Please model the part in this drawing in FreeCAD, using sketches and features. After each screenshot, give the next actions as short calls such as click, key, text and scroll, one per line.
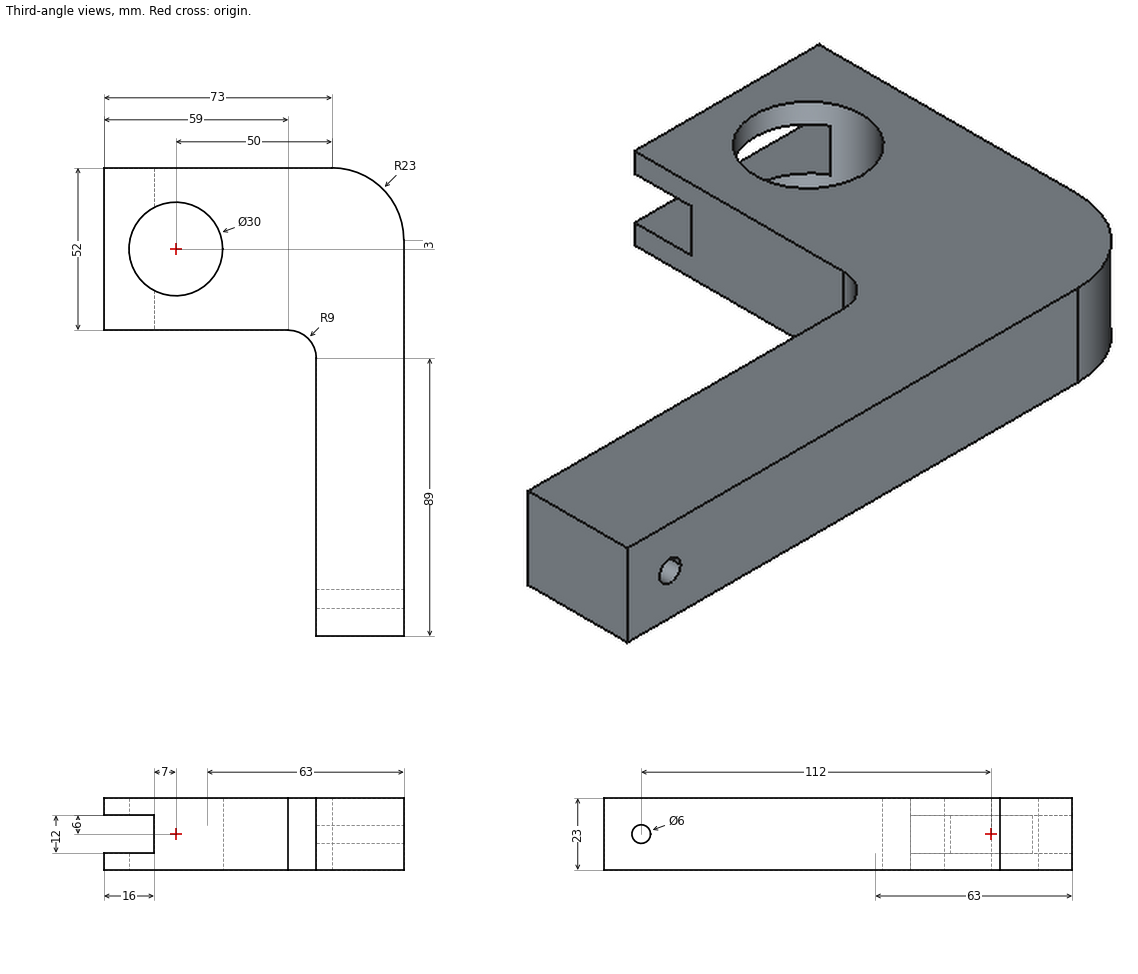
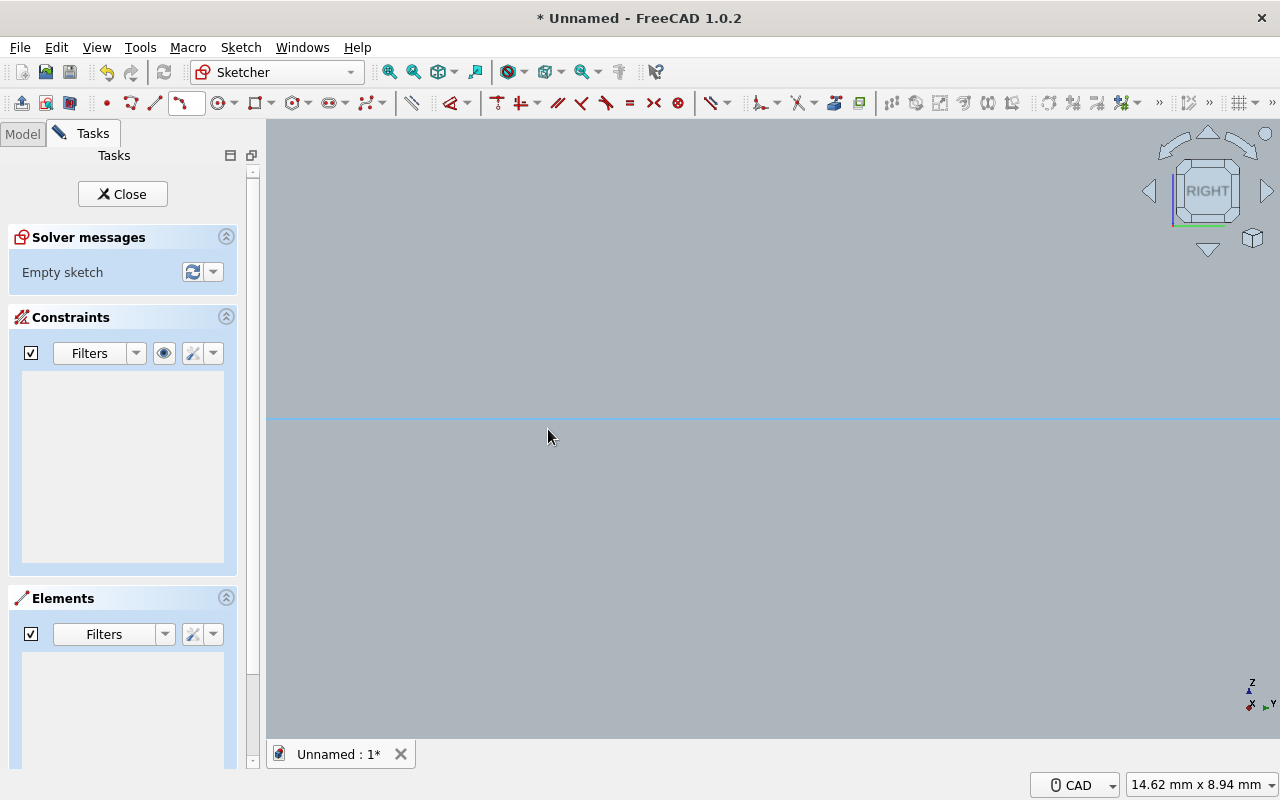
click(218, 104)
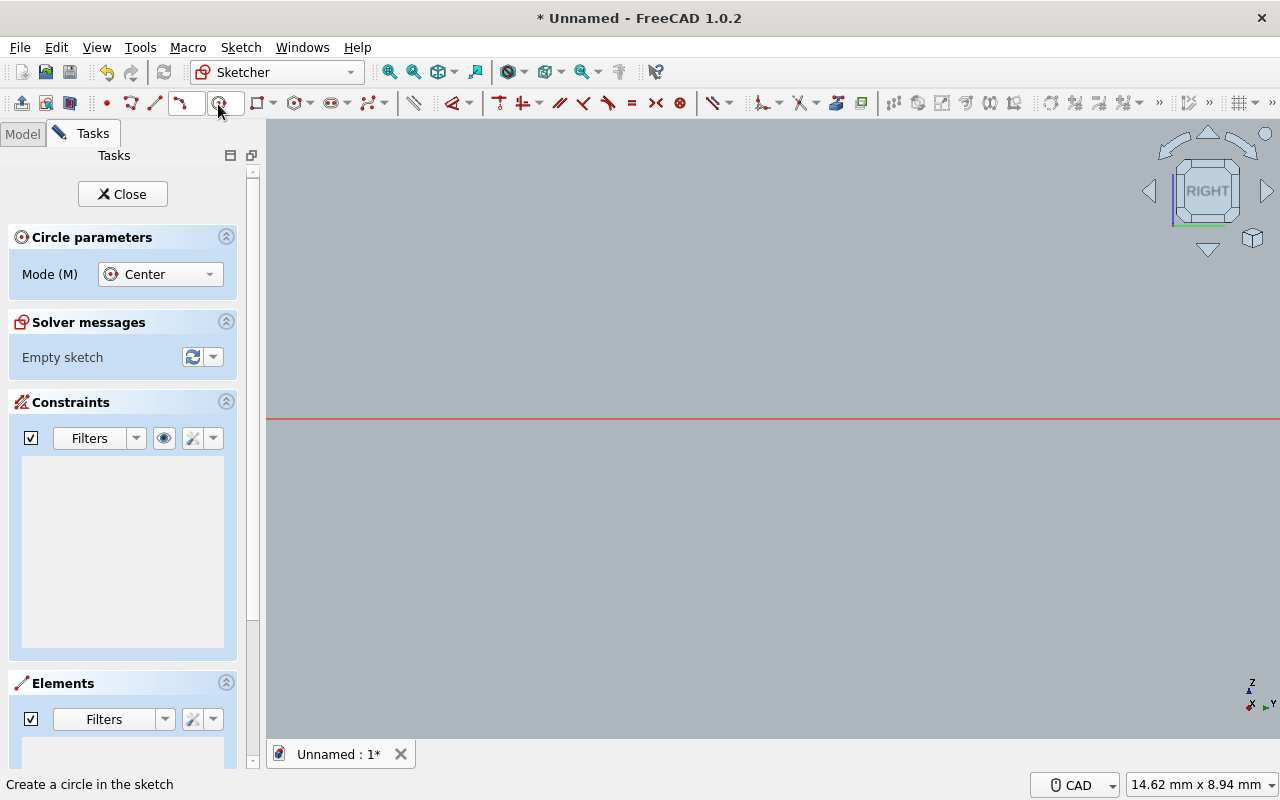
click(693, 419)
move(840, 272)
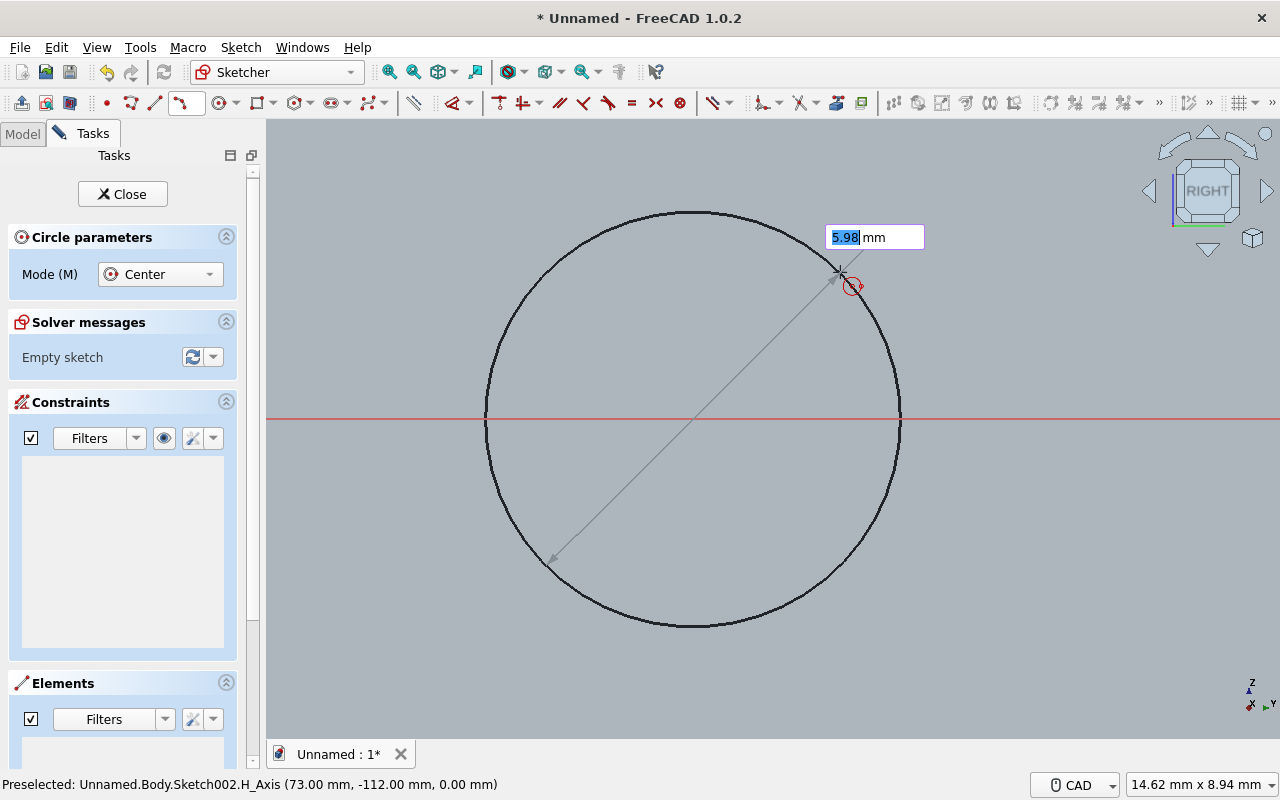
text(6)
key(Return)
key(Escape)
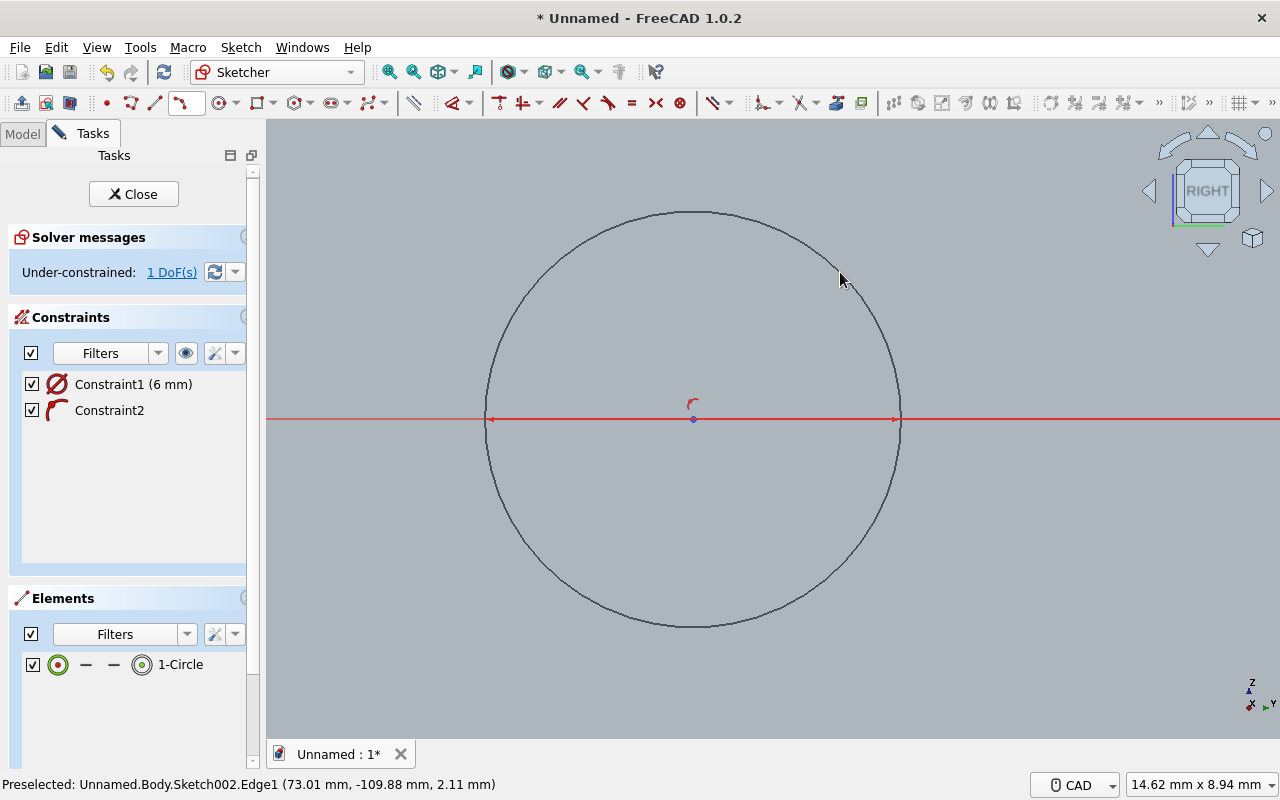
click(452, 104)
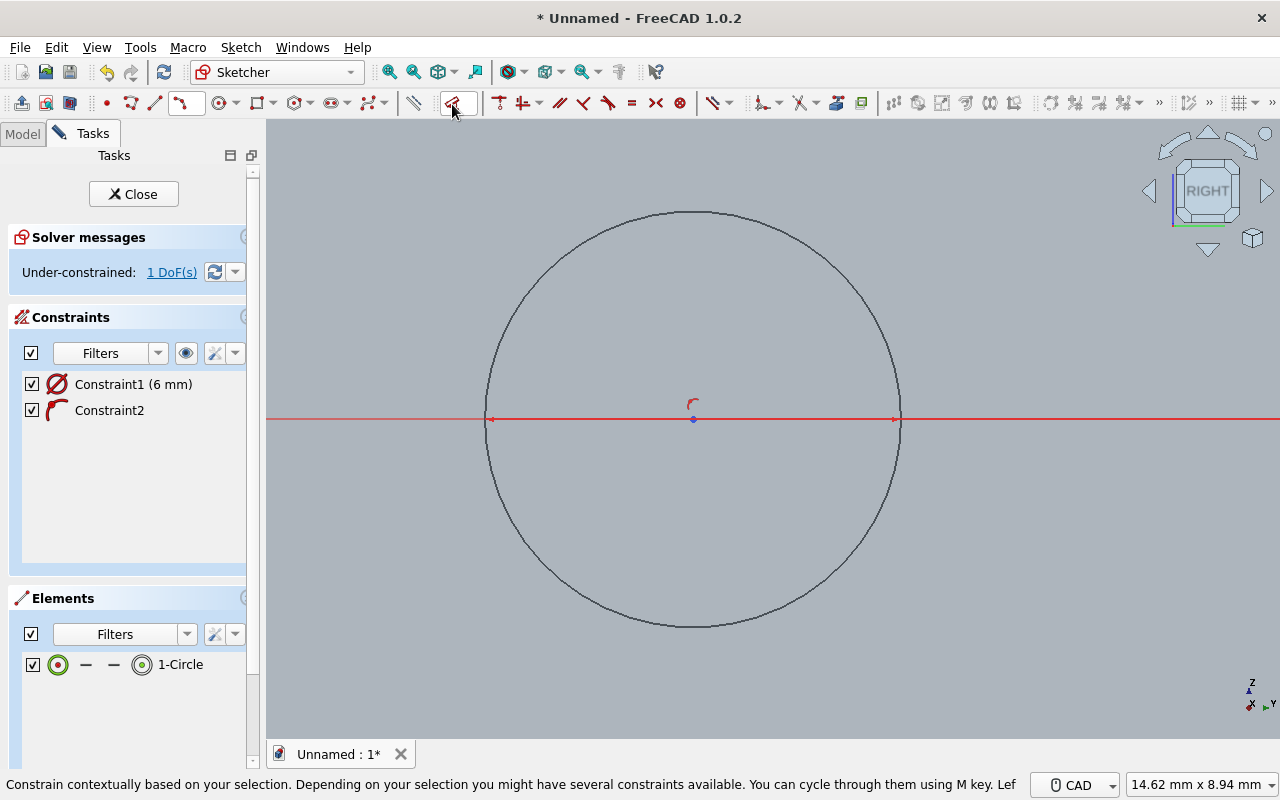
click(693, 419)
click(807, 453)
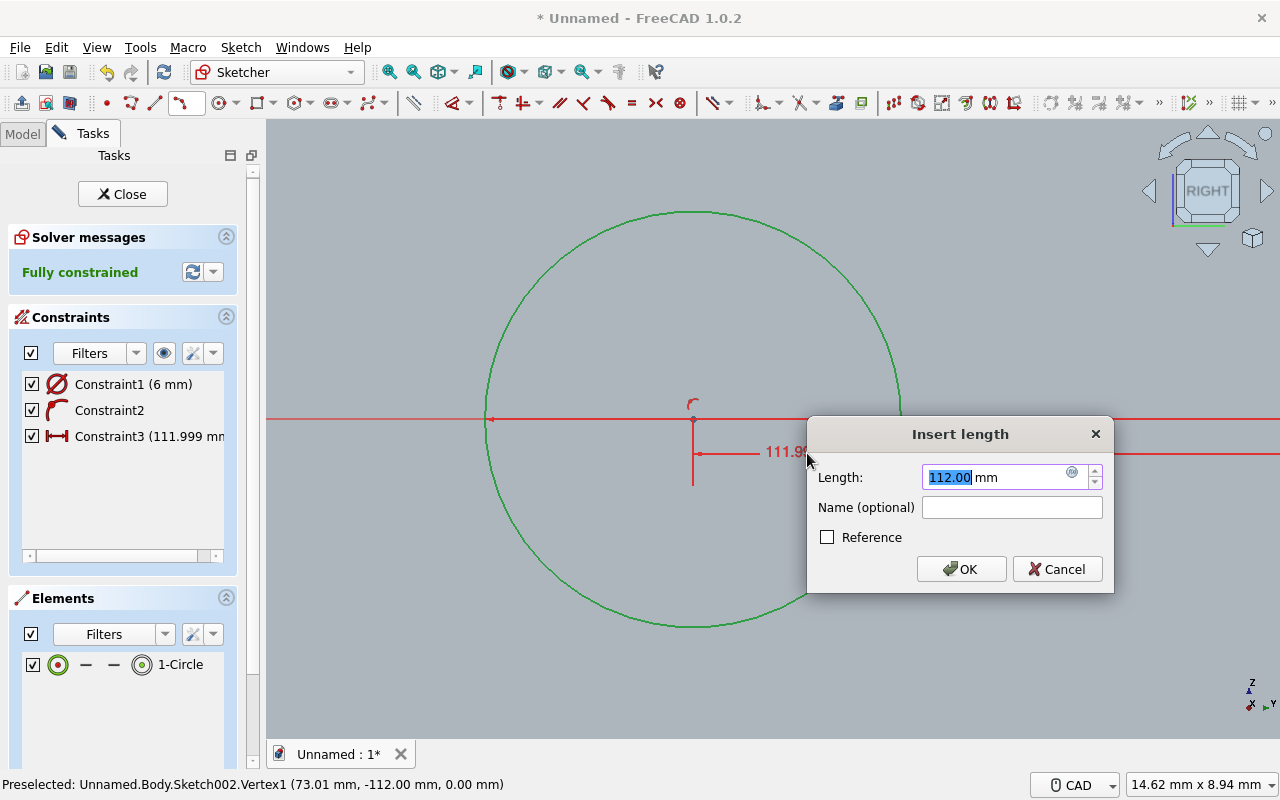
text(112)
key(Return)
key(Escape)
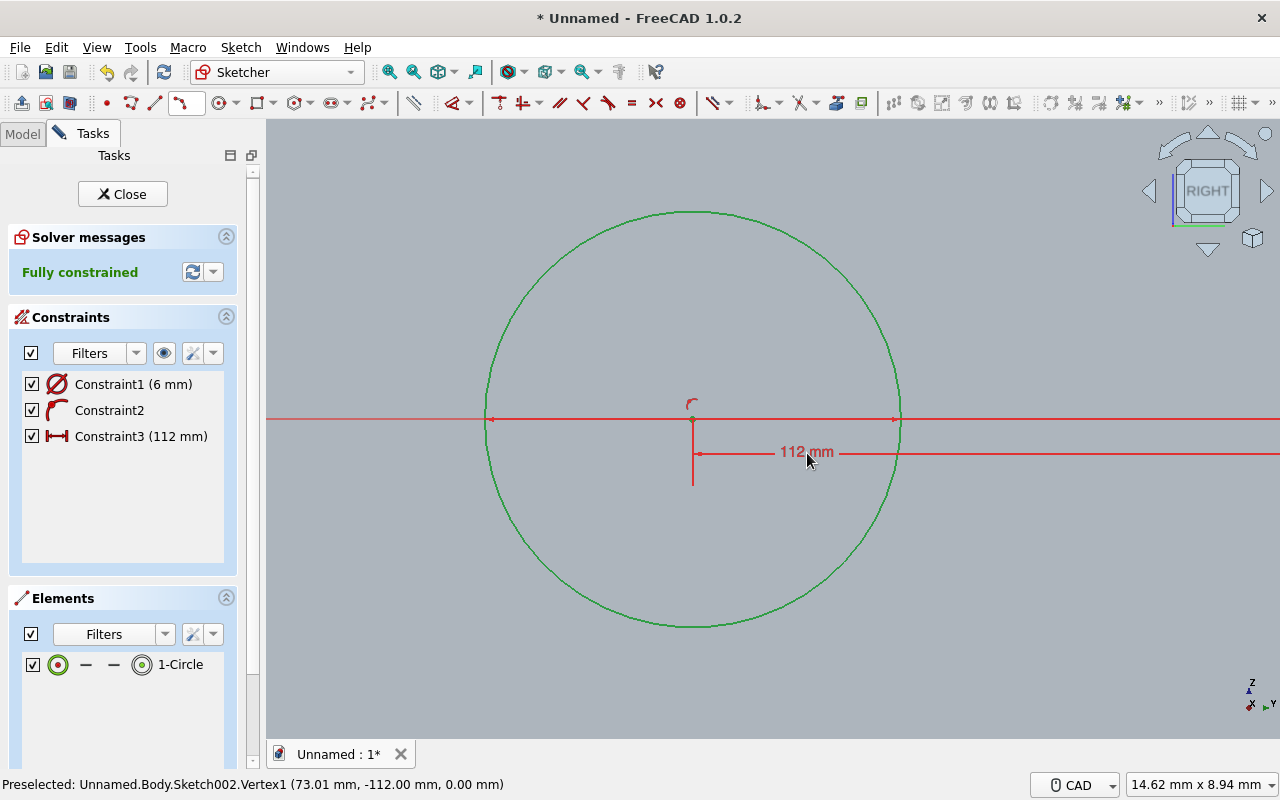
click(123, 194)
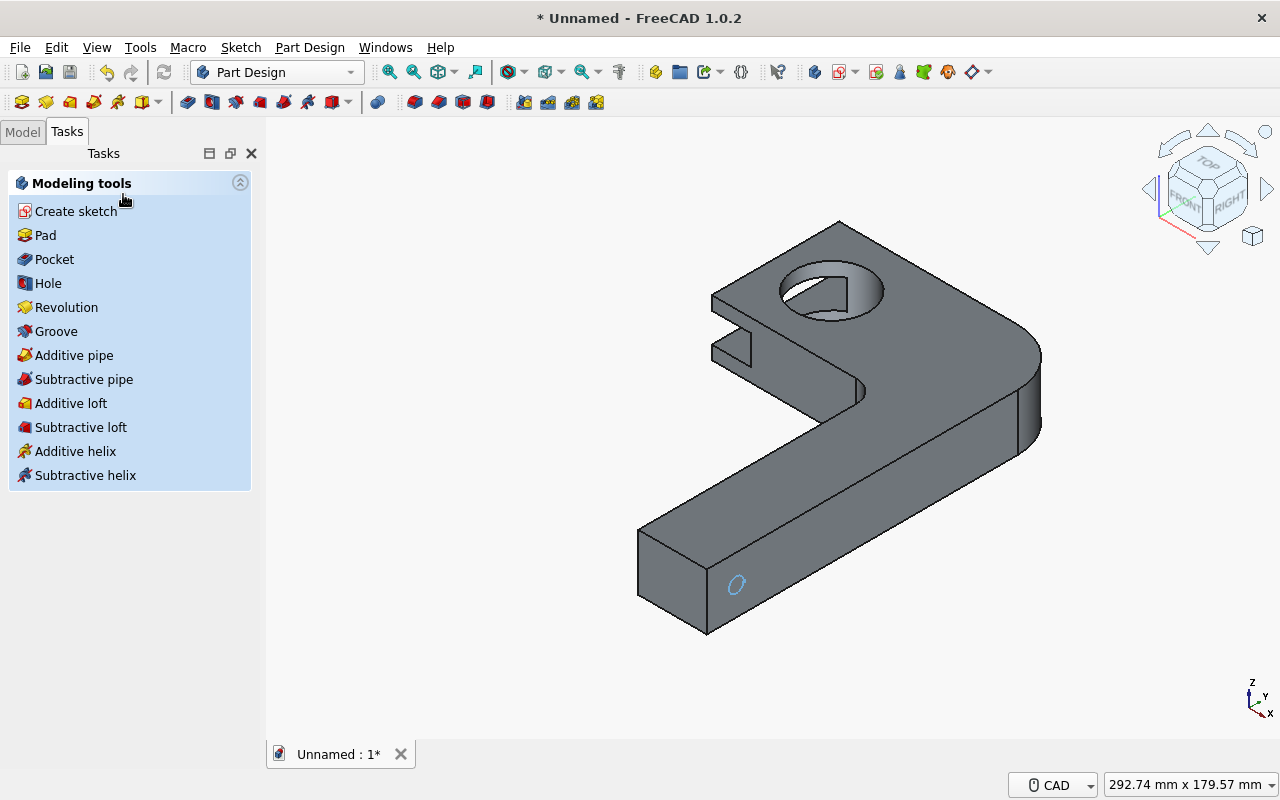
click(188, 102)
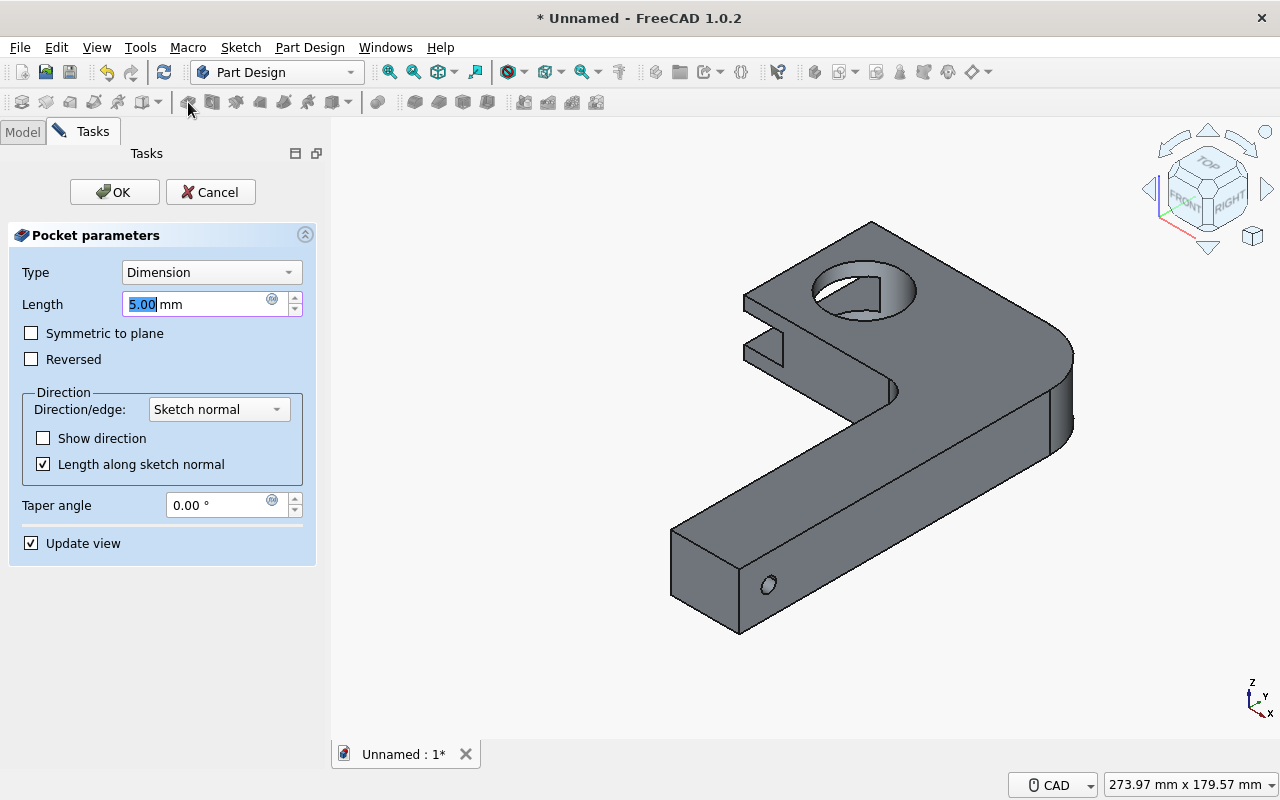
text(63)
key(Tab)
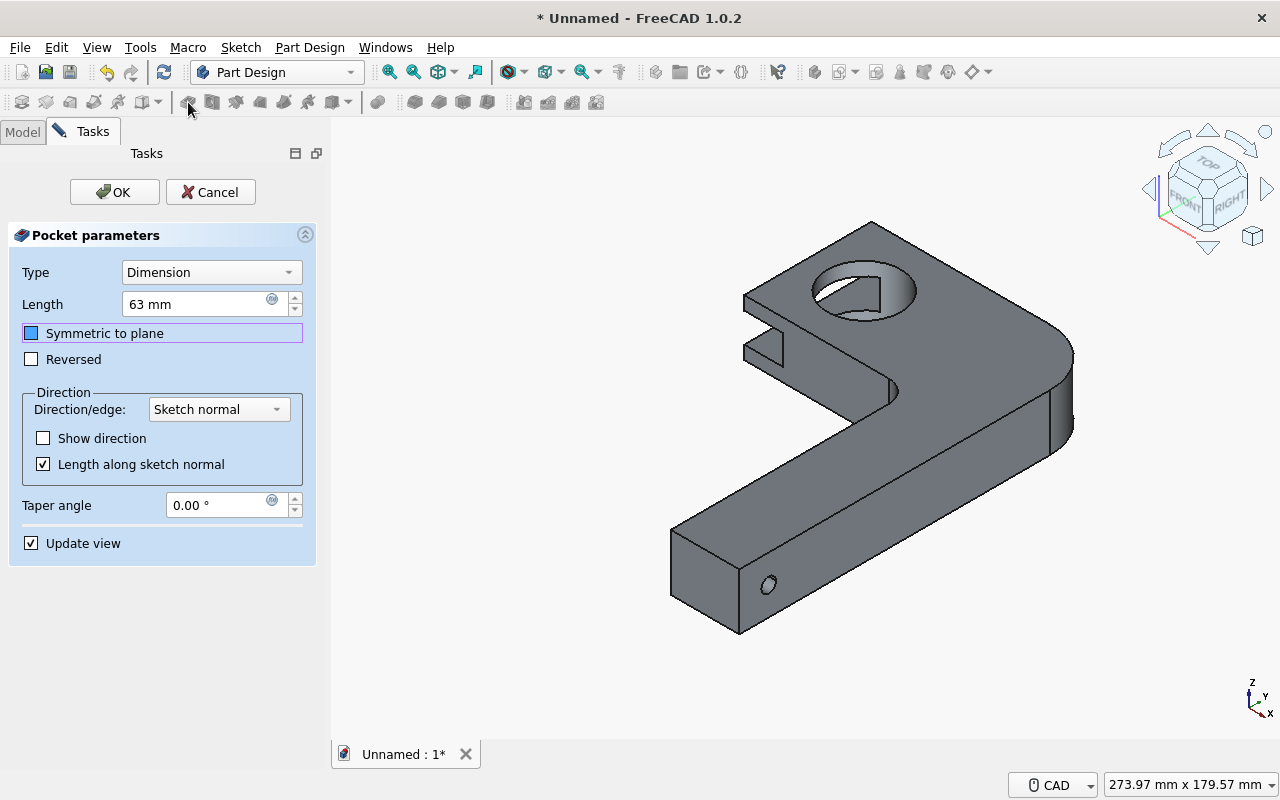
click(115, 192)